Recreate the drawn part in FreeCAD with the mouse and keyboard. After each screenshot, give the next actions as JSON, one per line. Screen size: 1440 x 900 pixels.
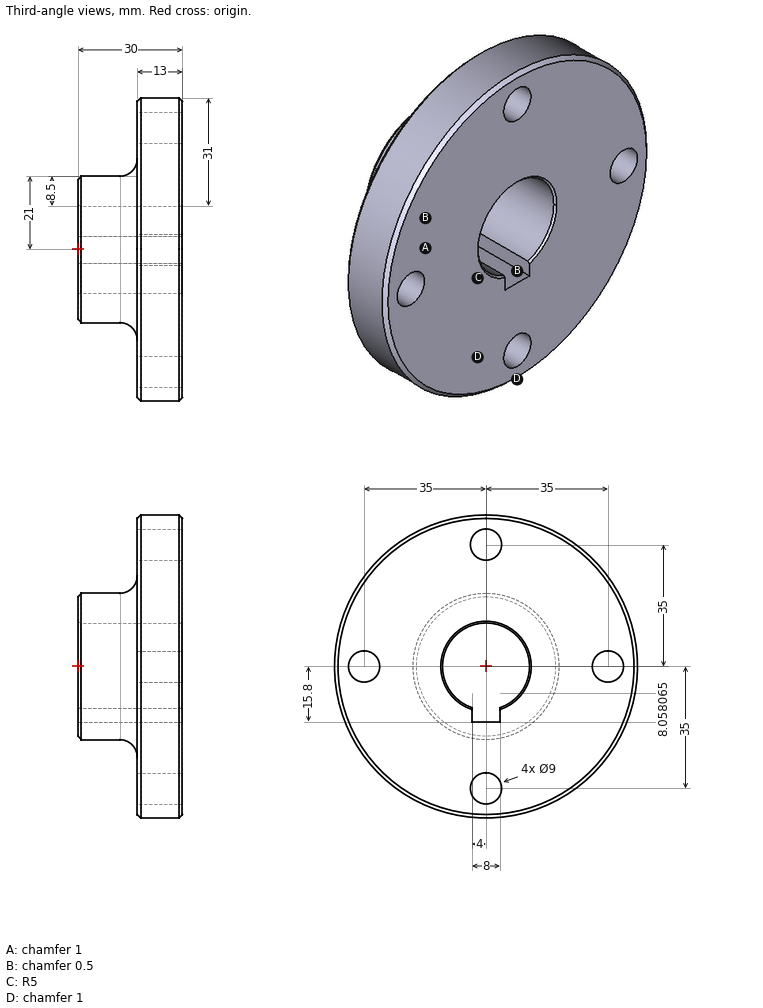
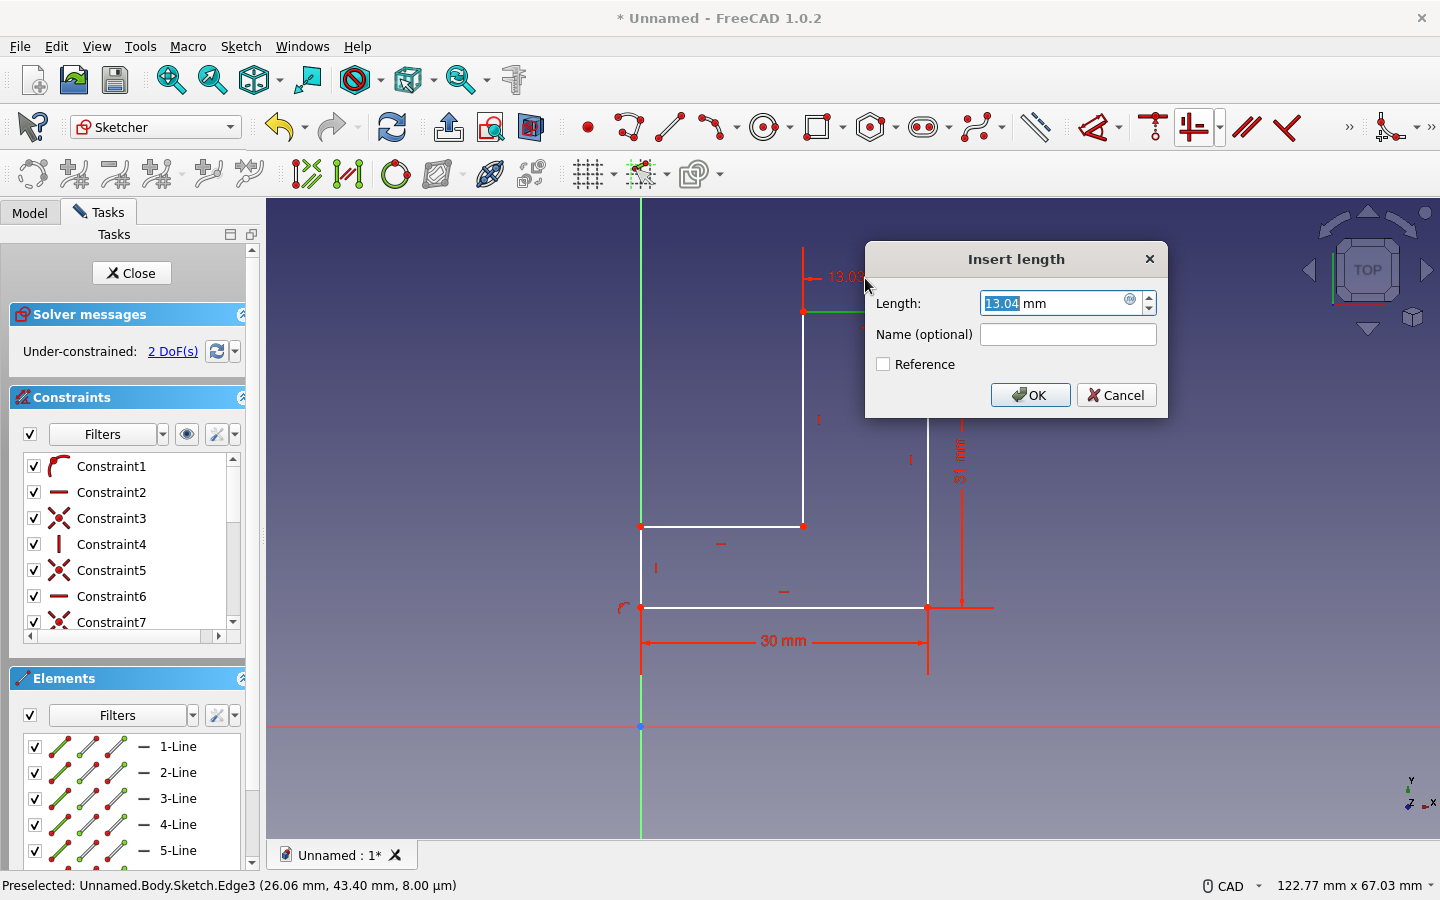
{"action": "type", "text": "13"}
{"action": "key", "text": "Return"}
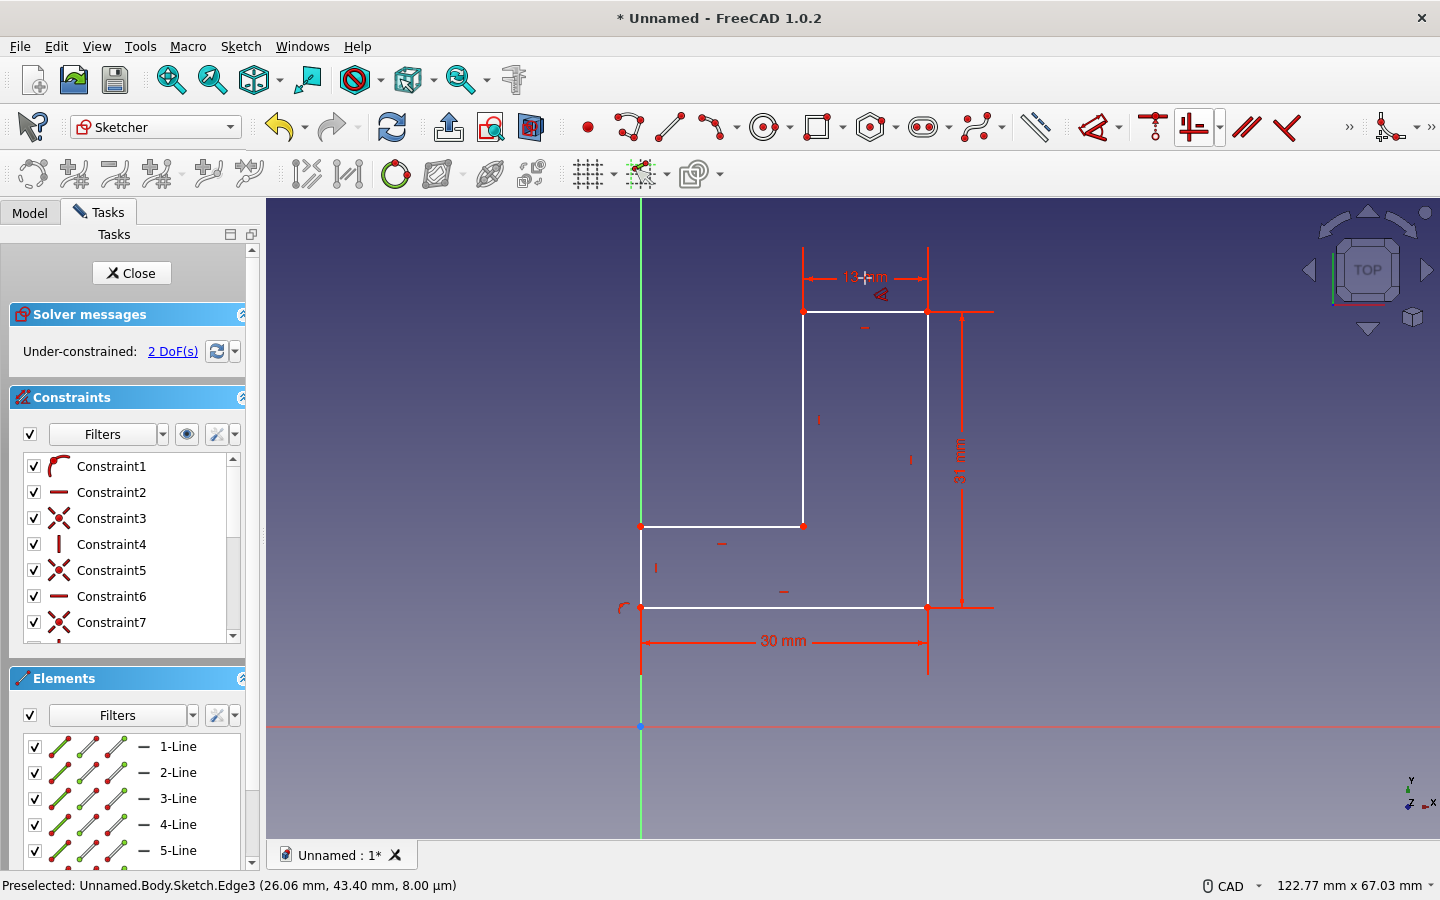
{"action": "left_click", "coordinate": [641, 551]}
{"action": "left_click", "coordinate": [607, 568]}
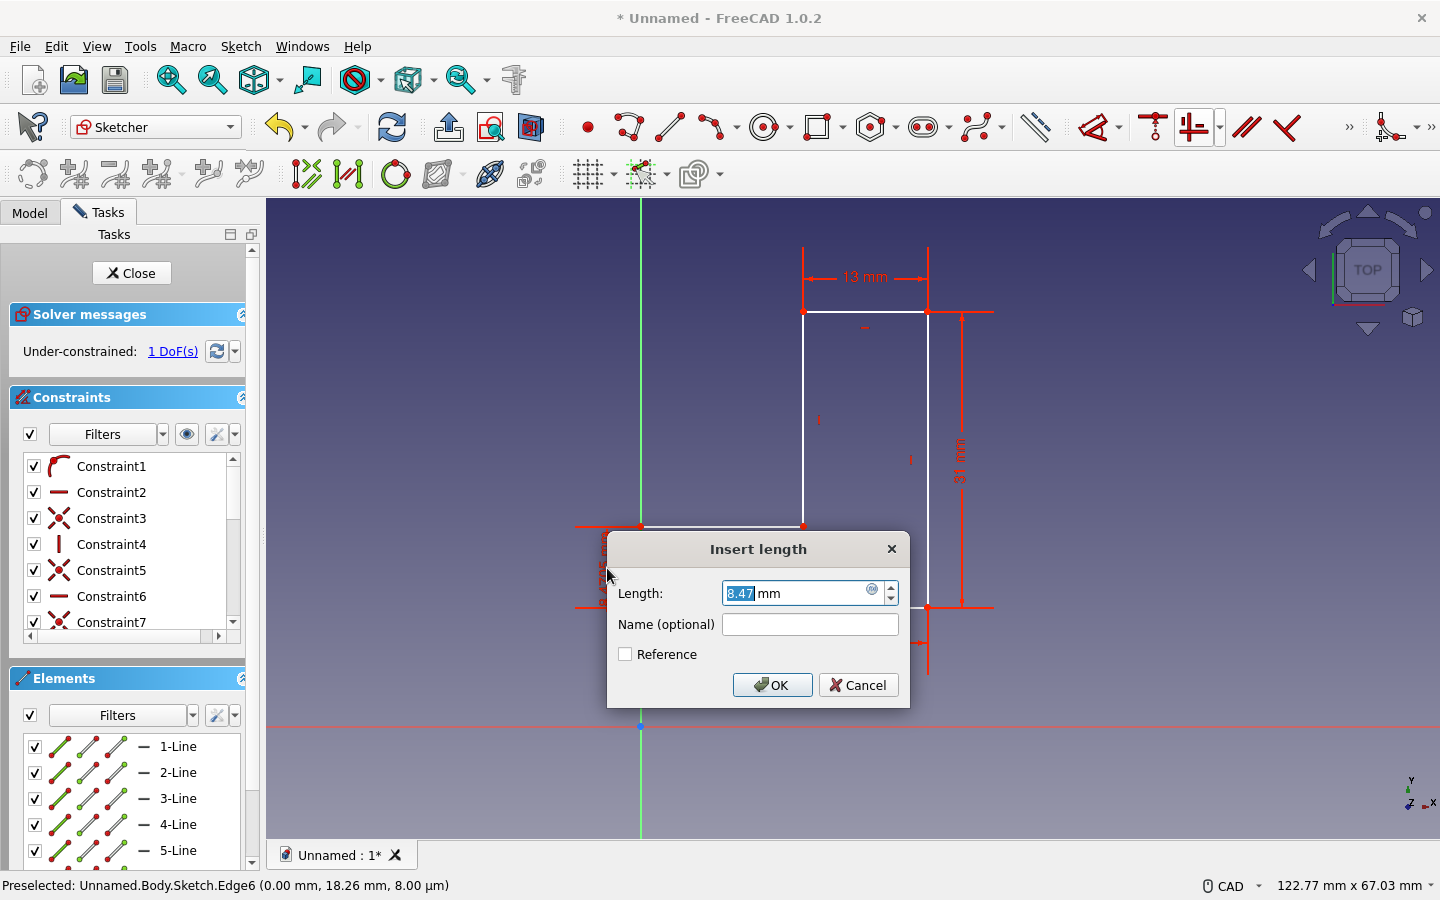
{"action": "type", "text": "8.5"}
{"action": "key", "text": "Return"}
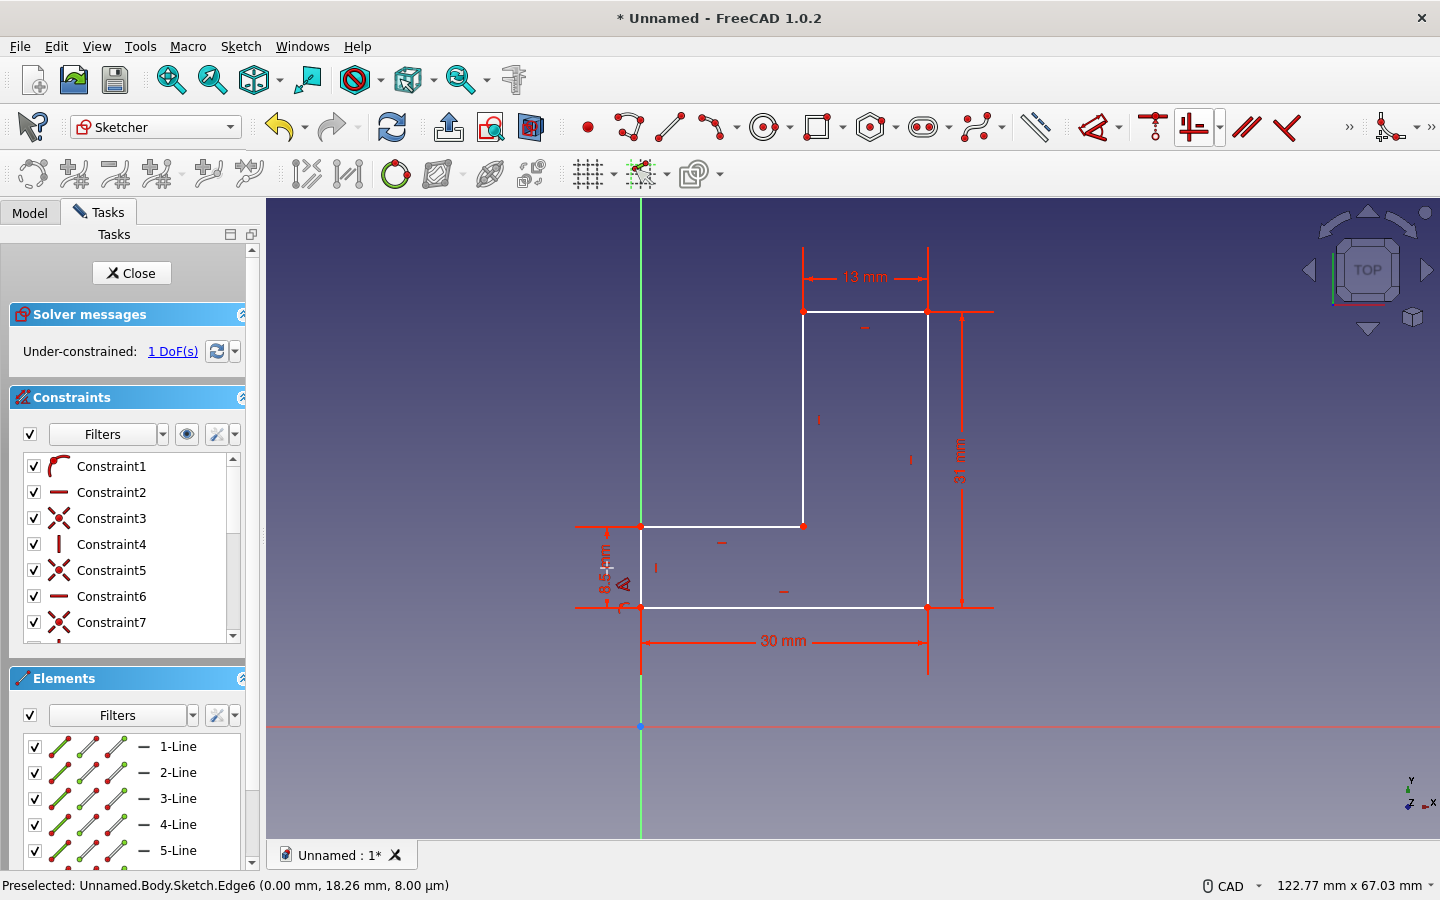
{"action": "left_click", "coordinate": [803, 527]}
{"action": "left_click", "coordinate": [607, 627]}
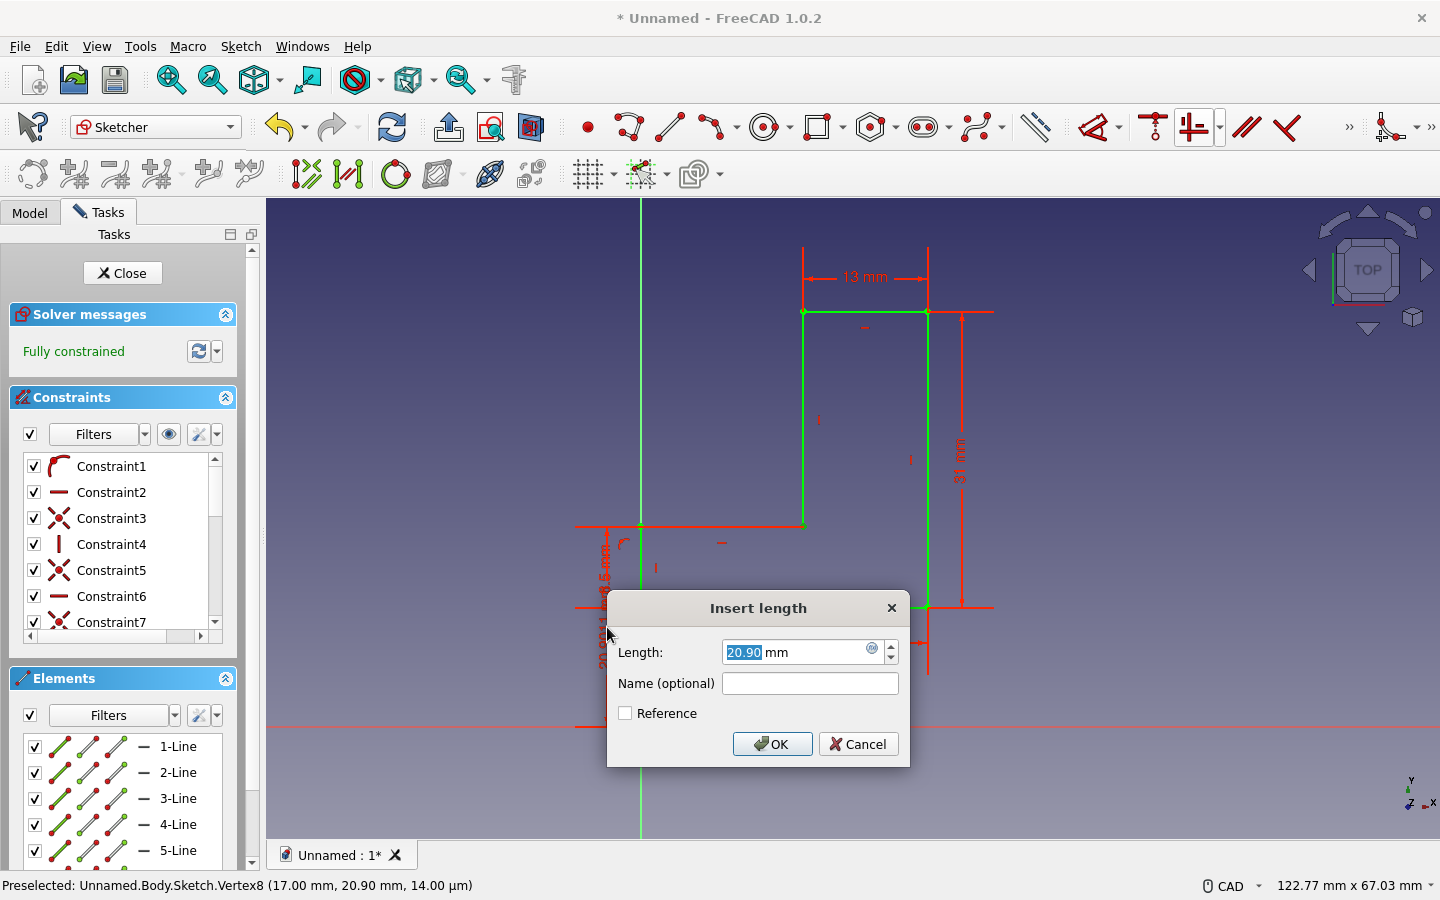
{"action": "type", "text": "21"}
{"action": "key", "text": "Return"}
{"action": "key", "text": "Escape"}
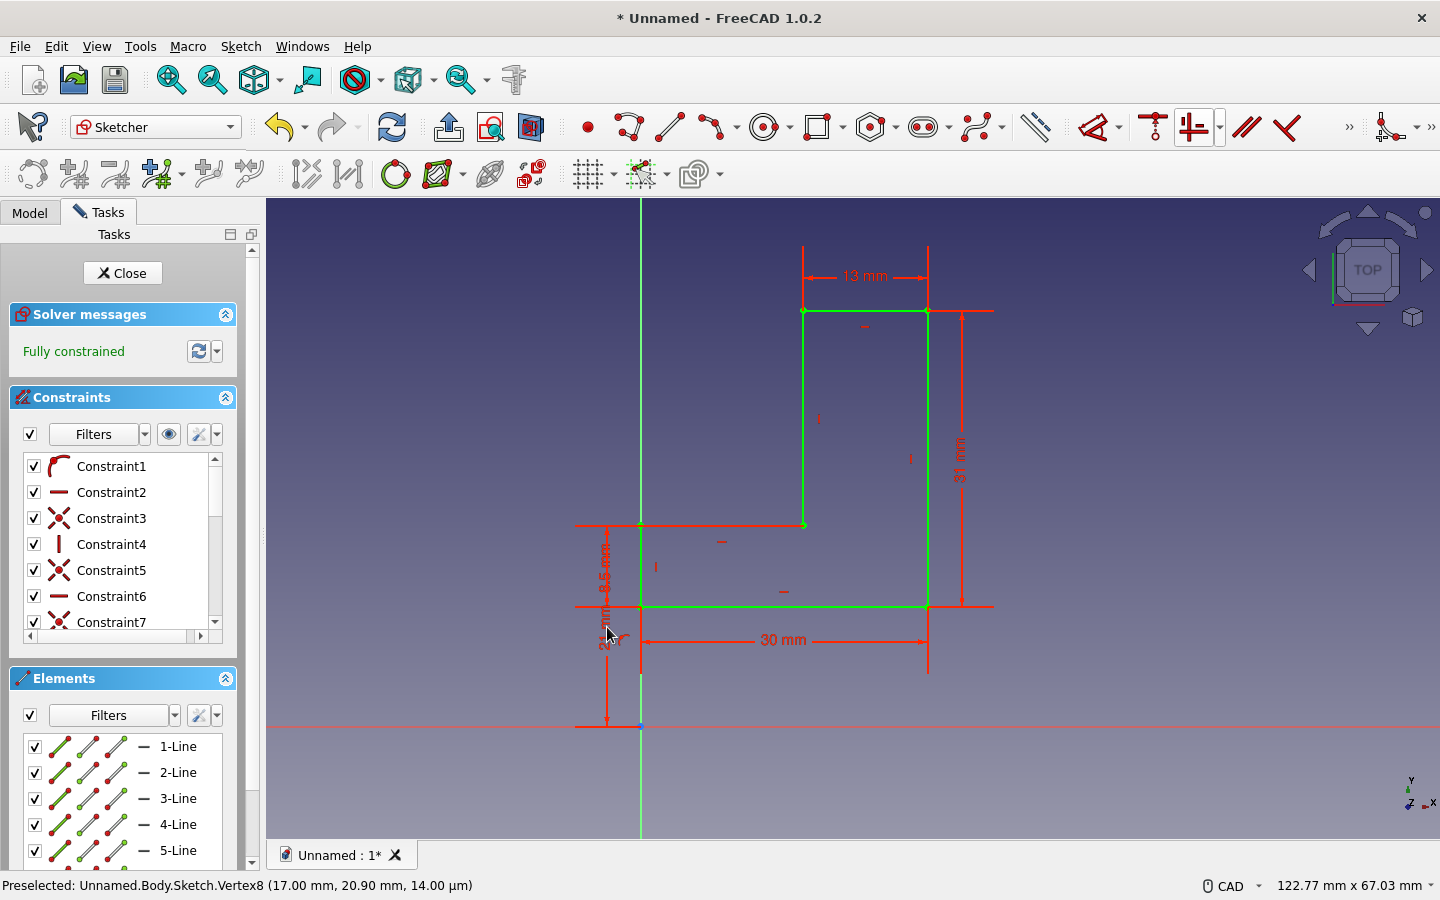
{"action": "left_click", "coordinate": [123, 273]}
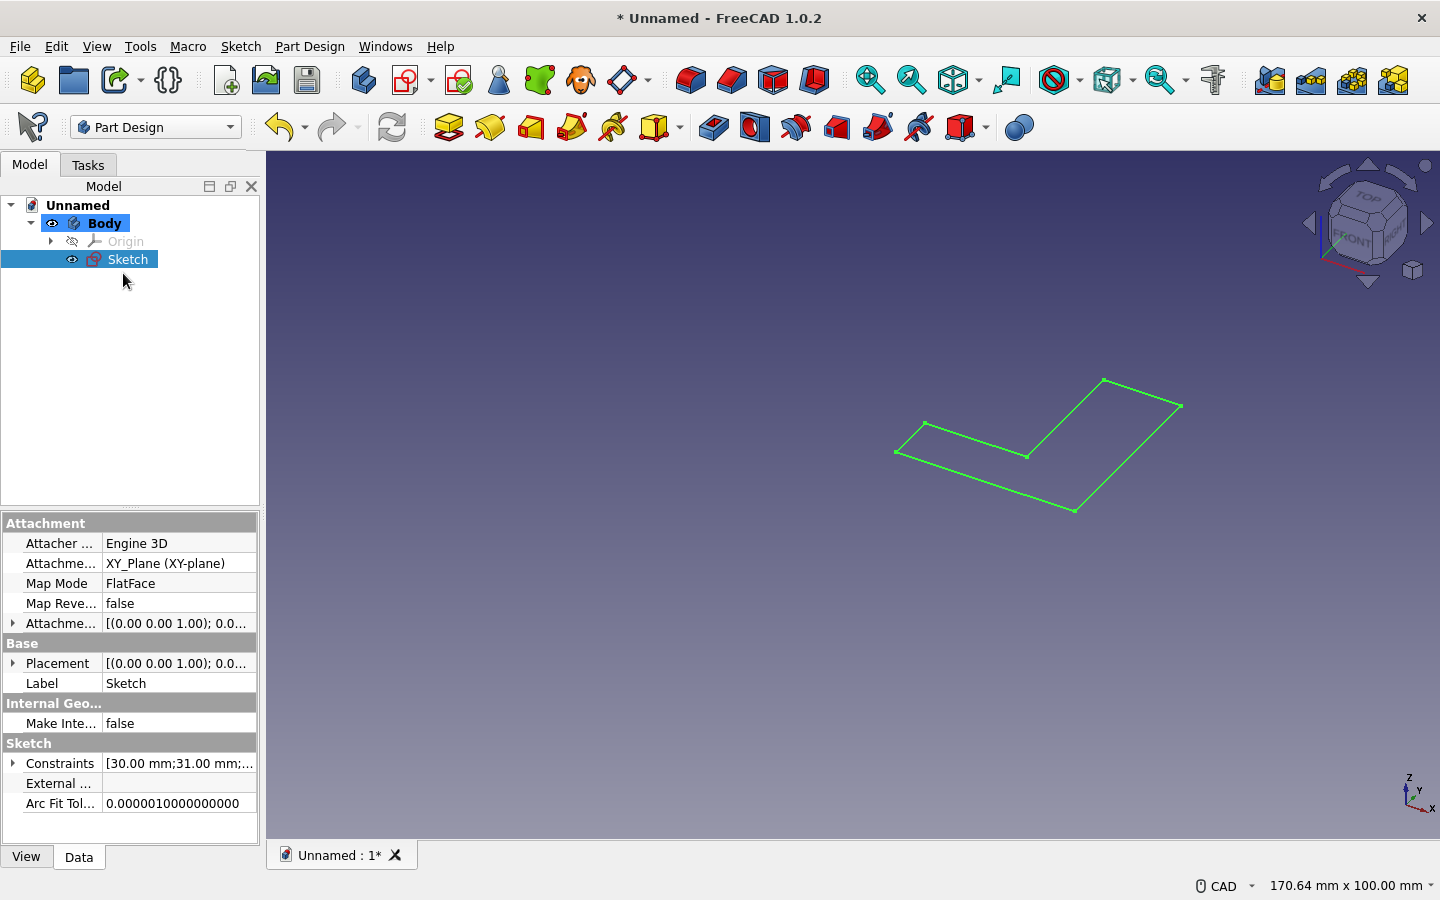
{"action": "left_click", "coordinate": [490, 128]}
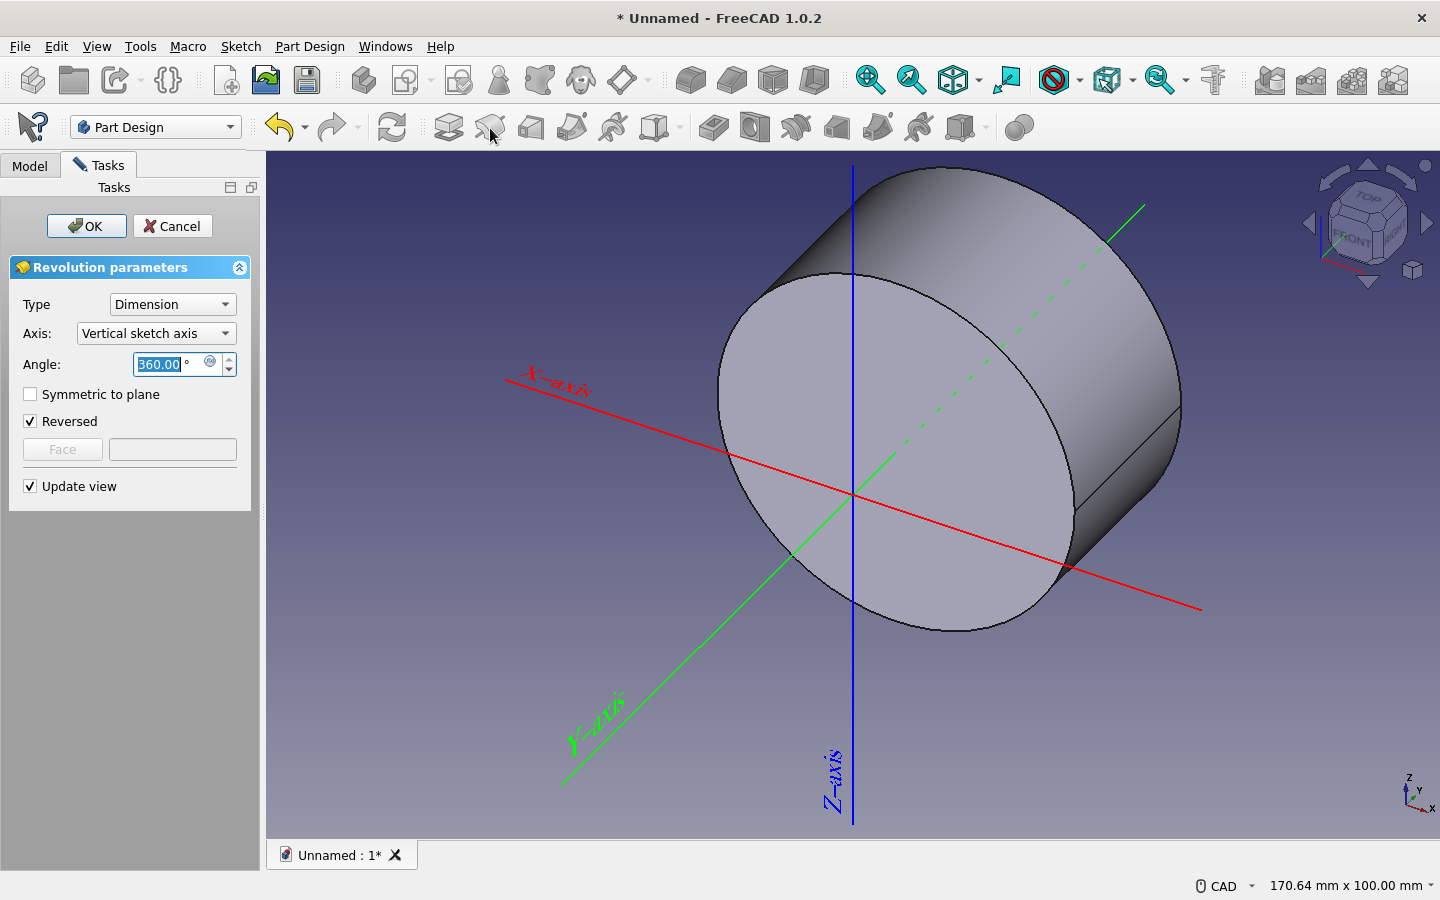
{"action": "left_click", "coordinate": [157, 334]}